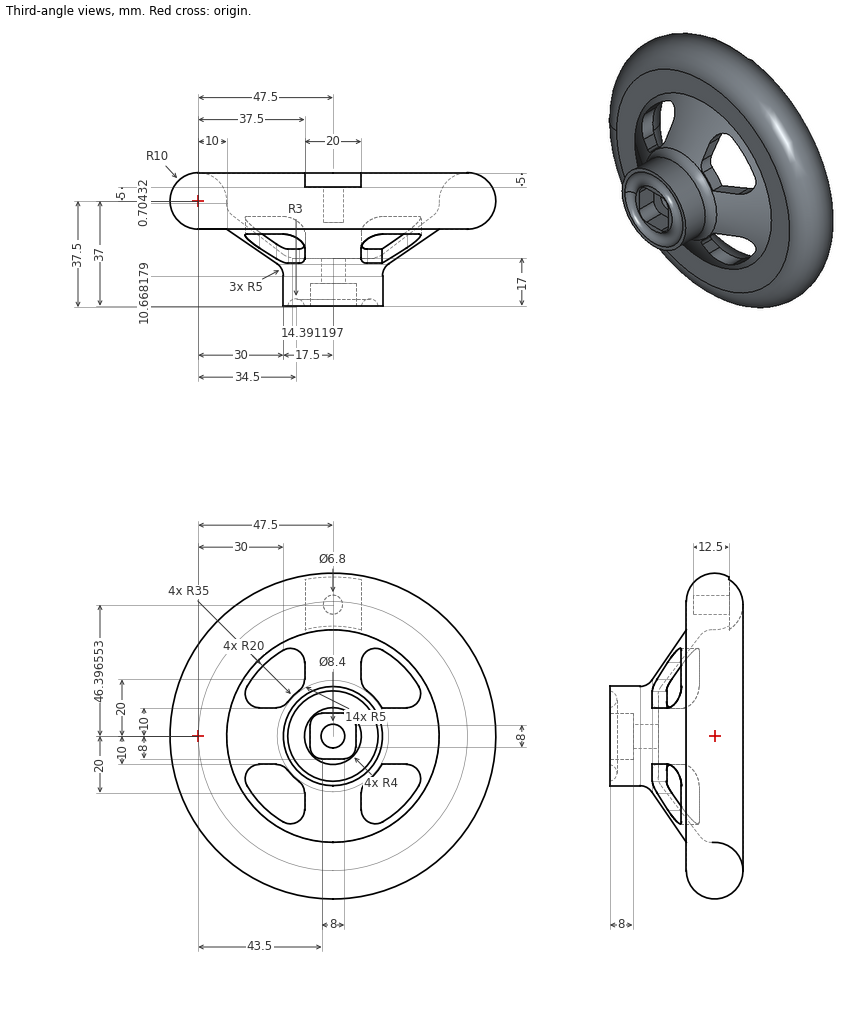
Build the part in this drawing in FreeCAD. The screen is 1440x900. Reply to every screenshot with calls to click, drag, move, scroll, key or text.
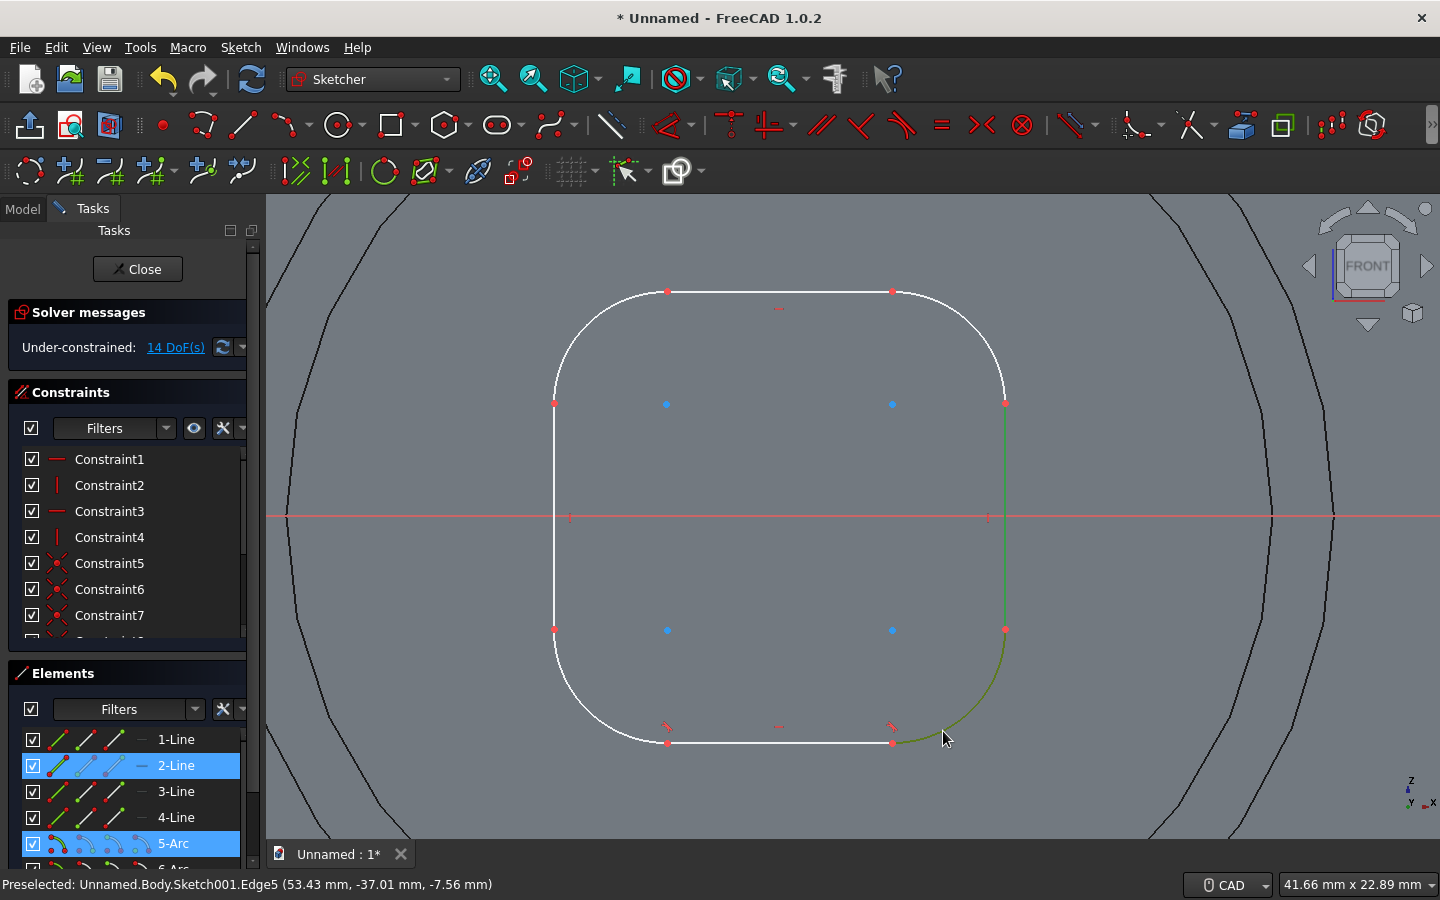
click(902, 126)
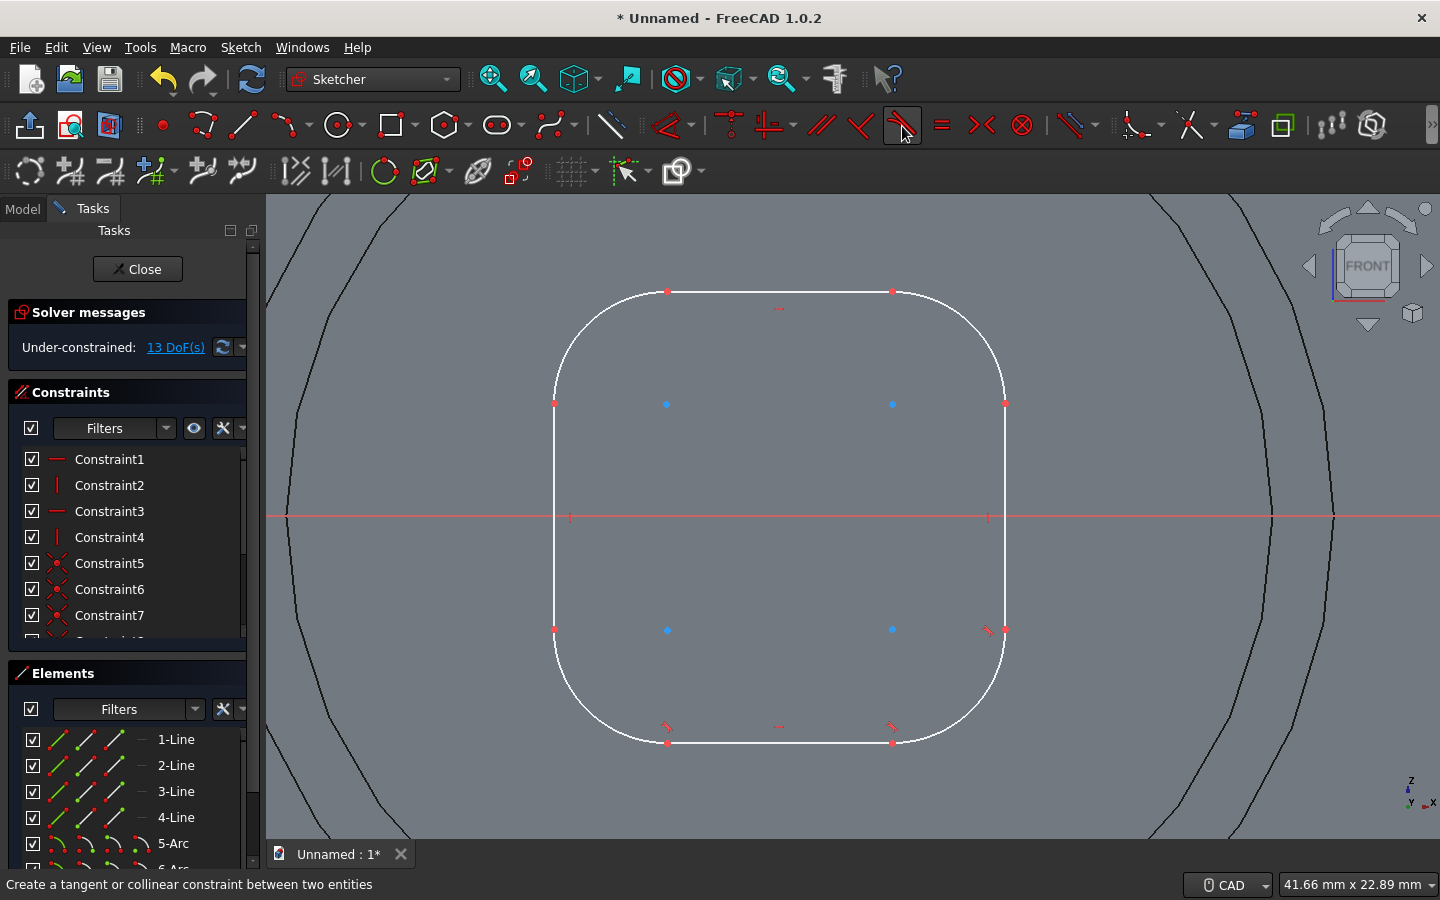
click(1005, 562)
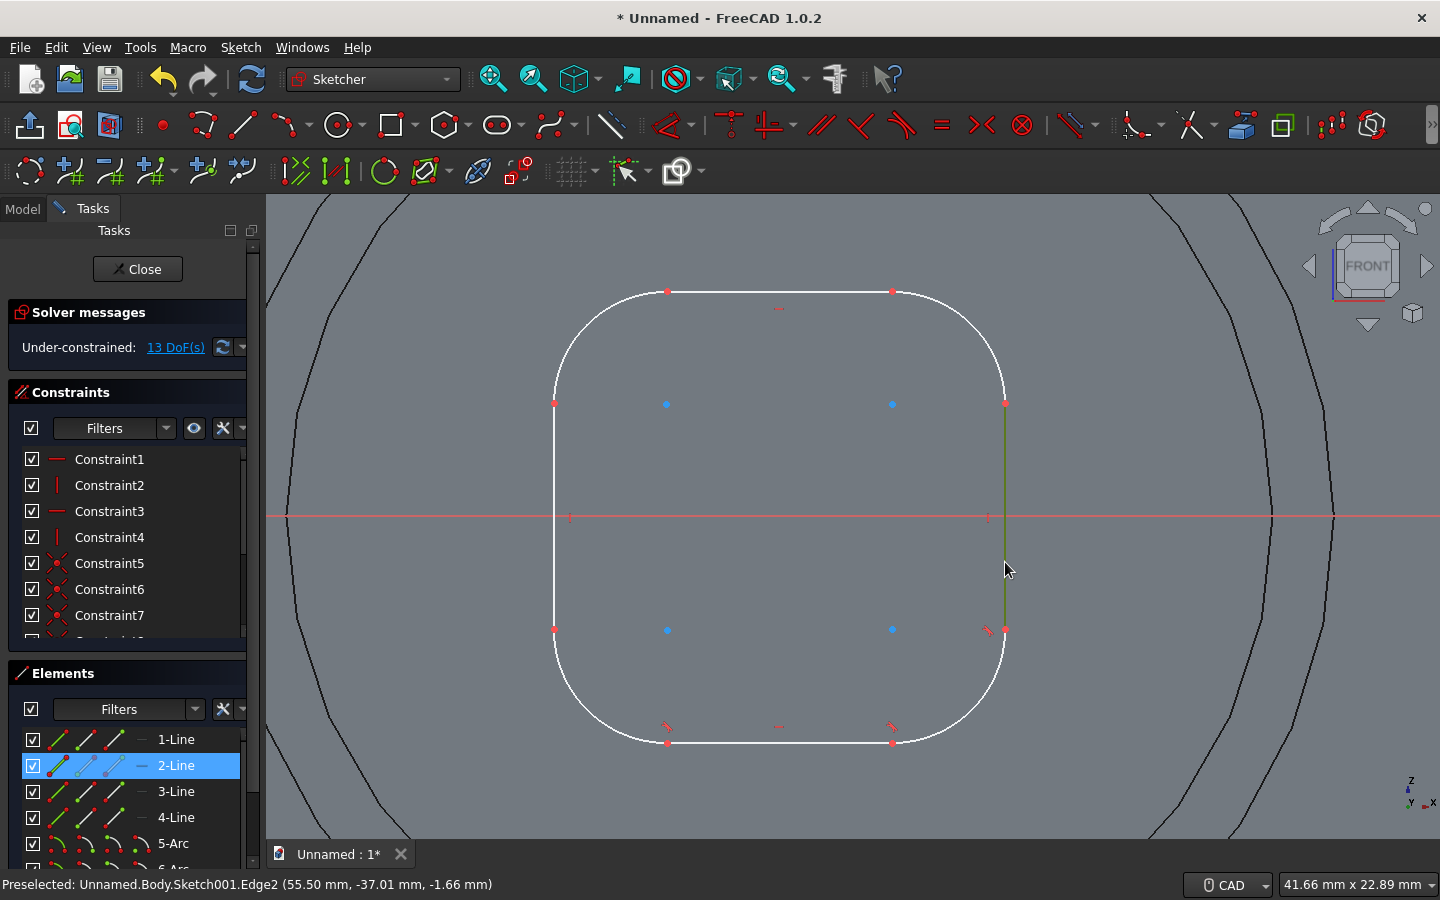
click(992, 353)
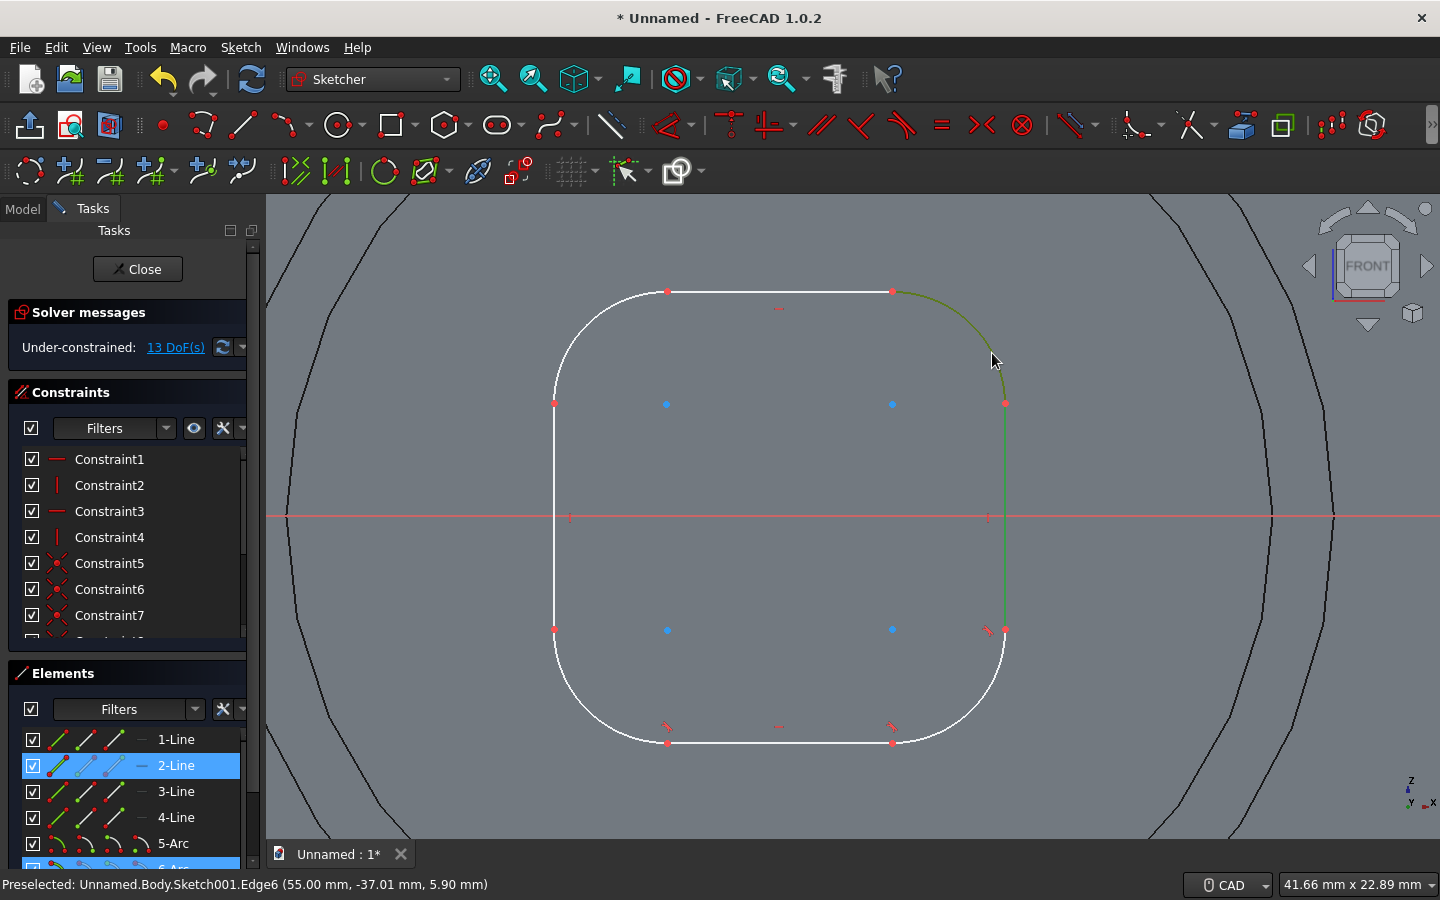
click(902, 126)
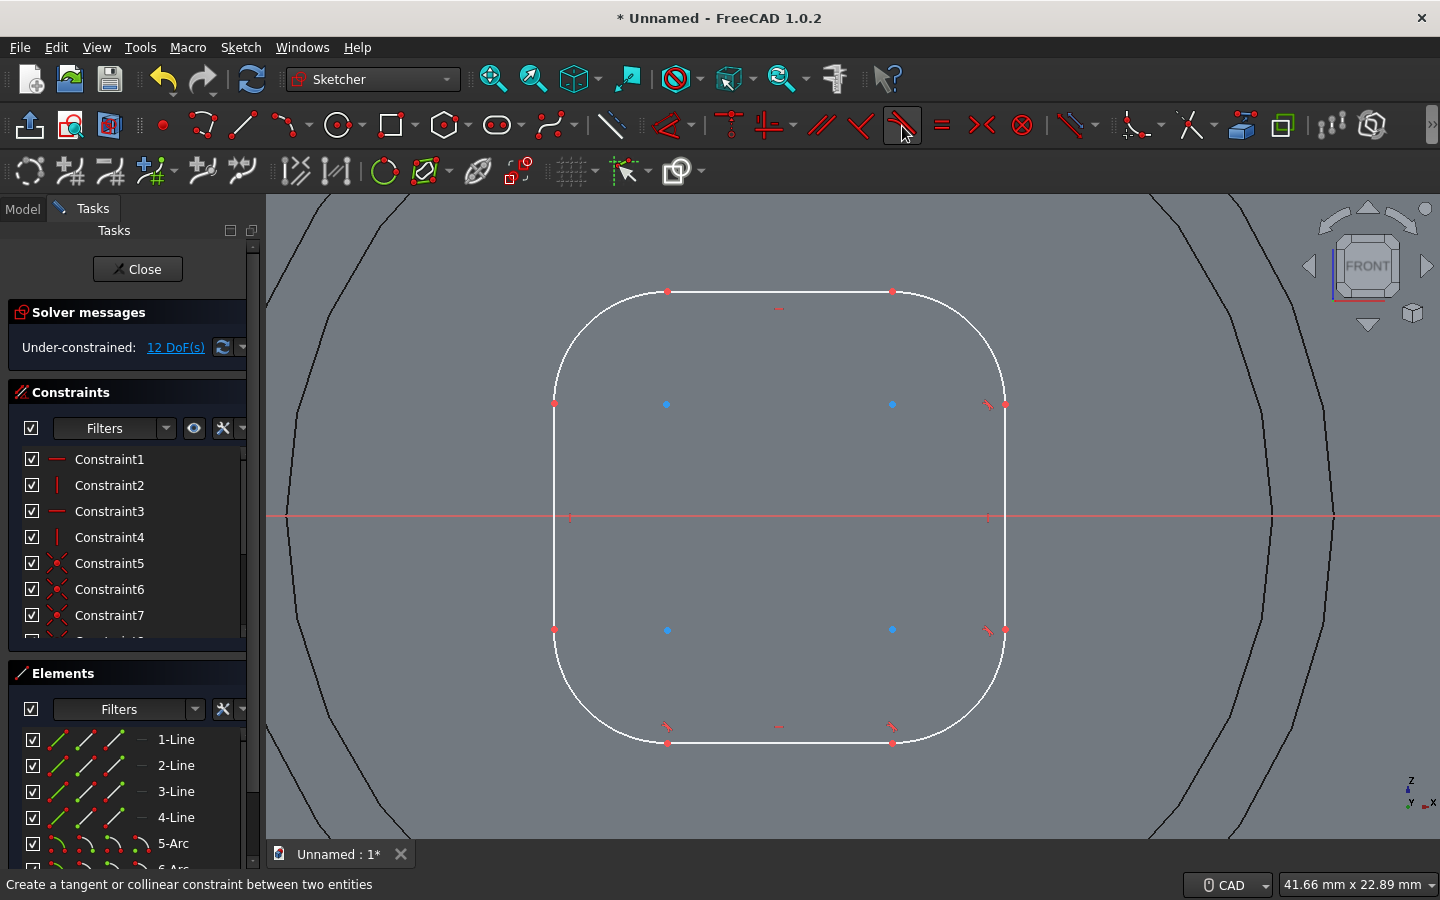
click(824, 292)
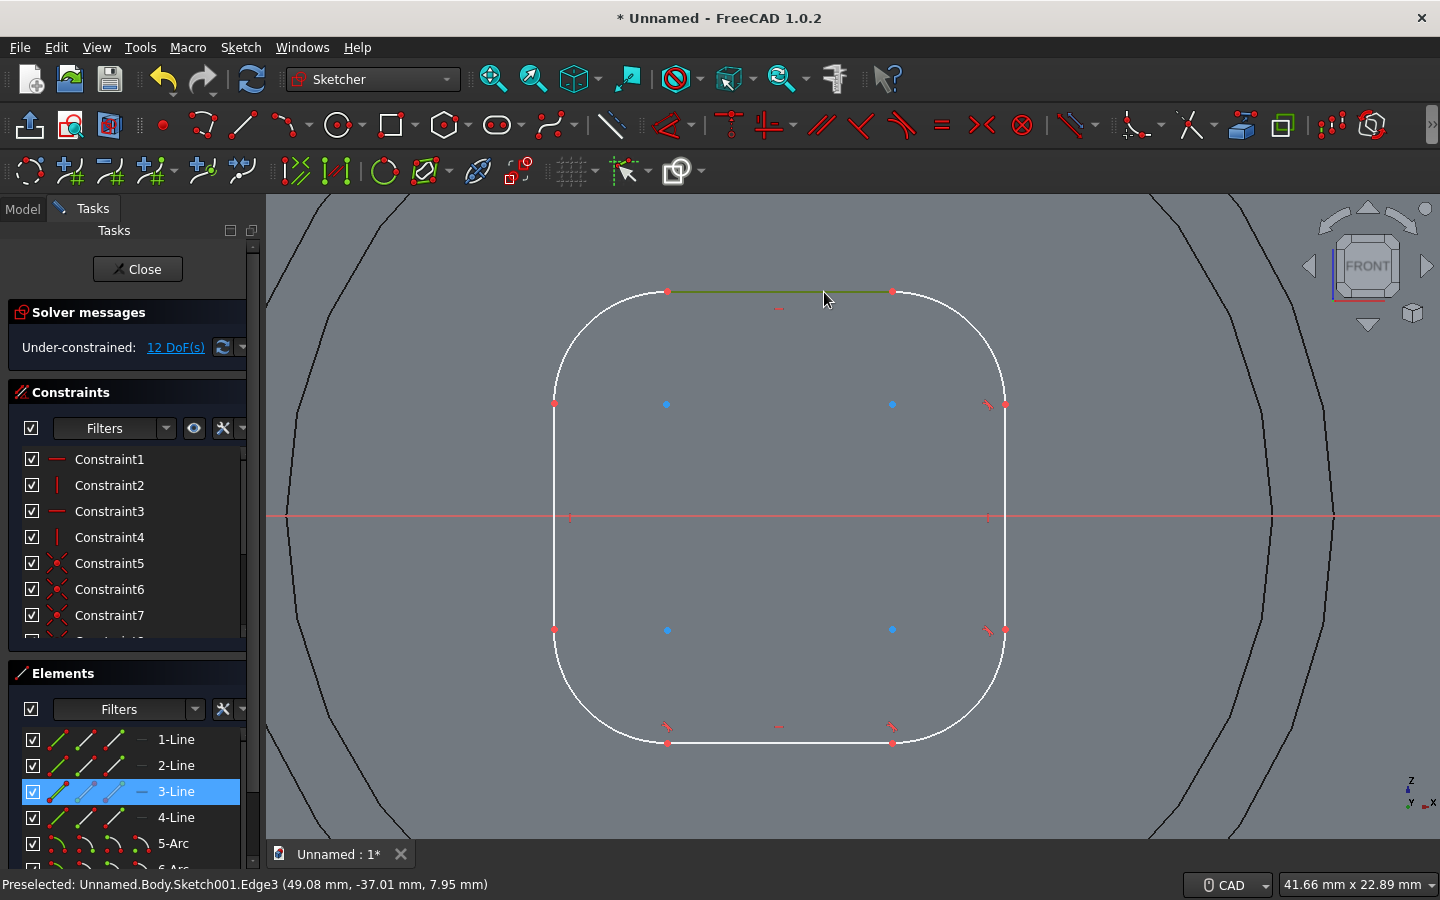
click(993, 353)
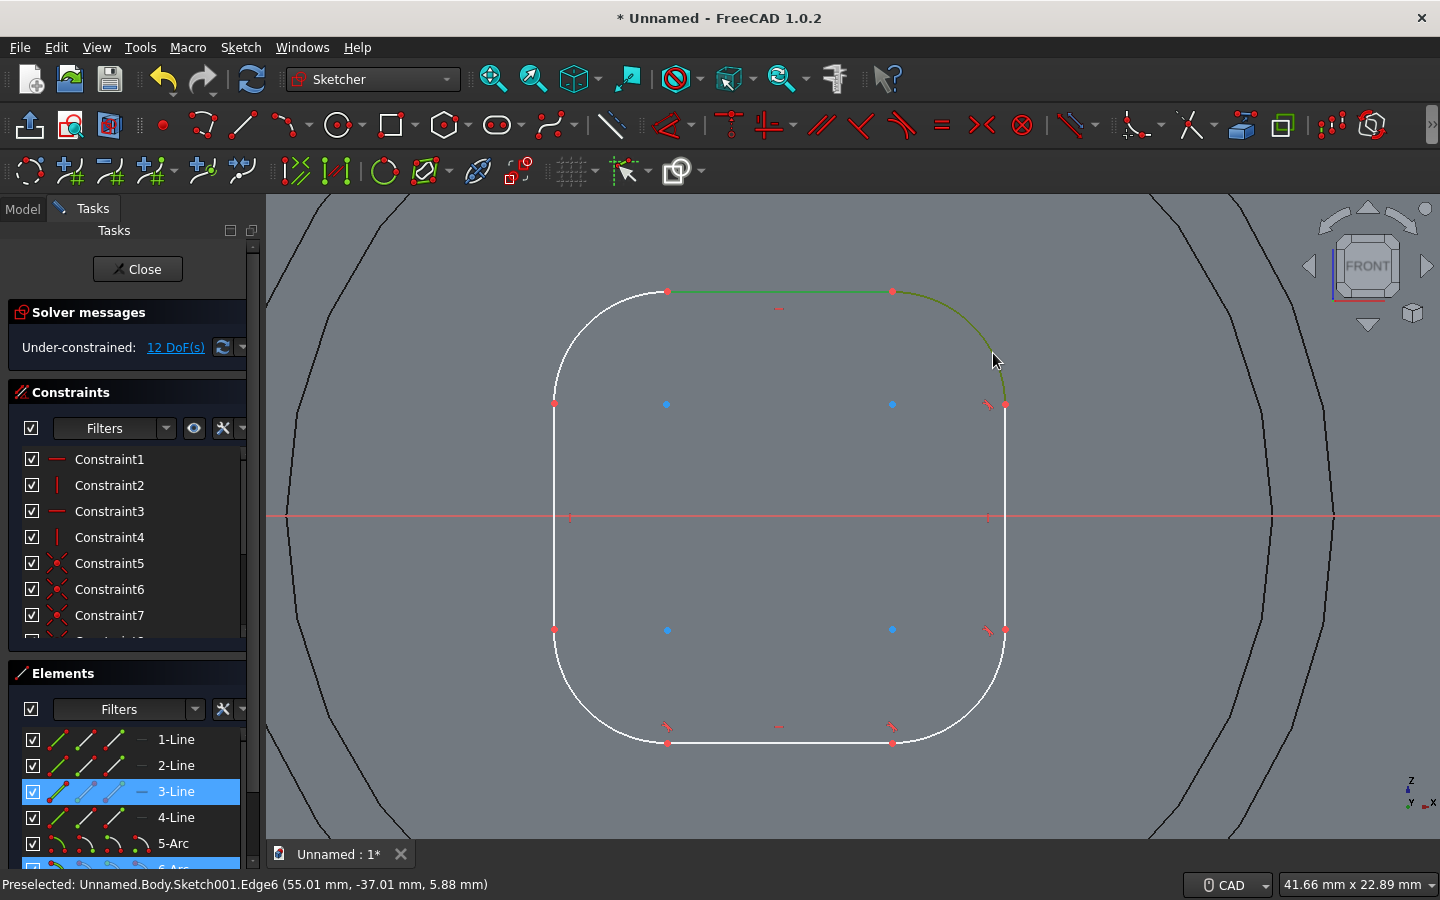
click(902, 126)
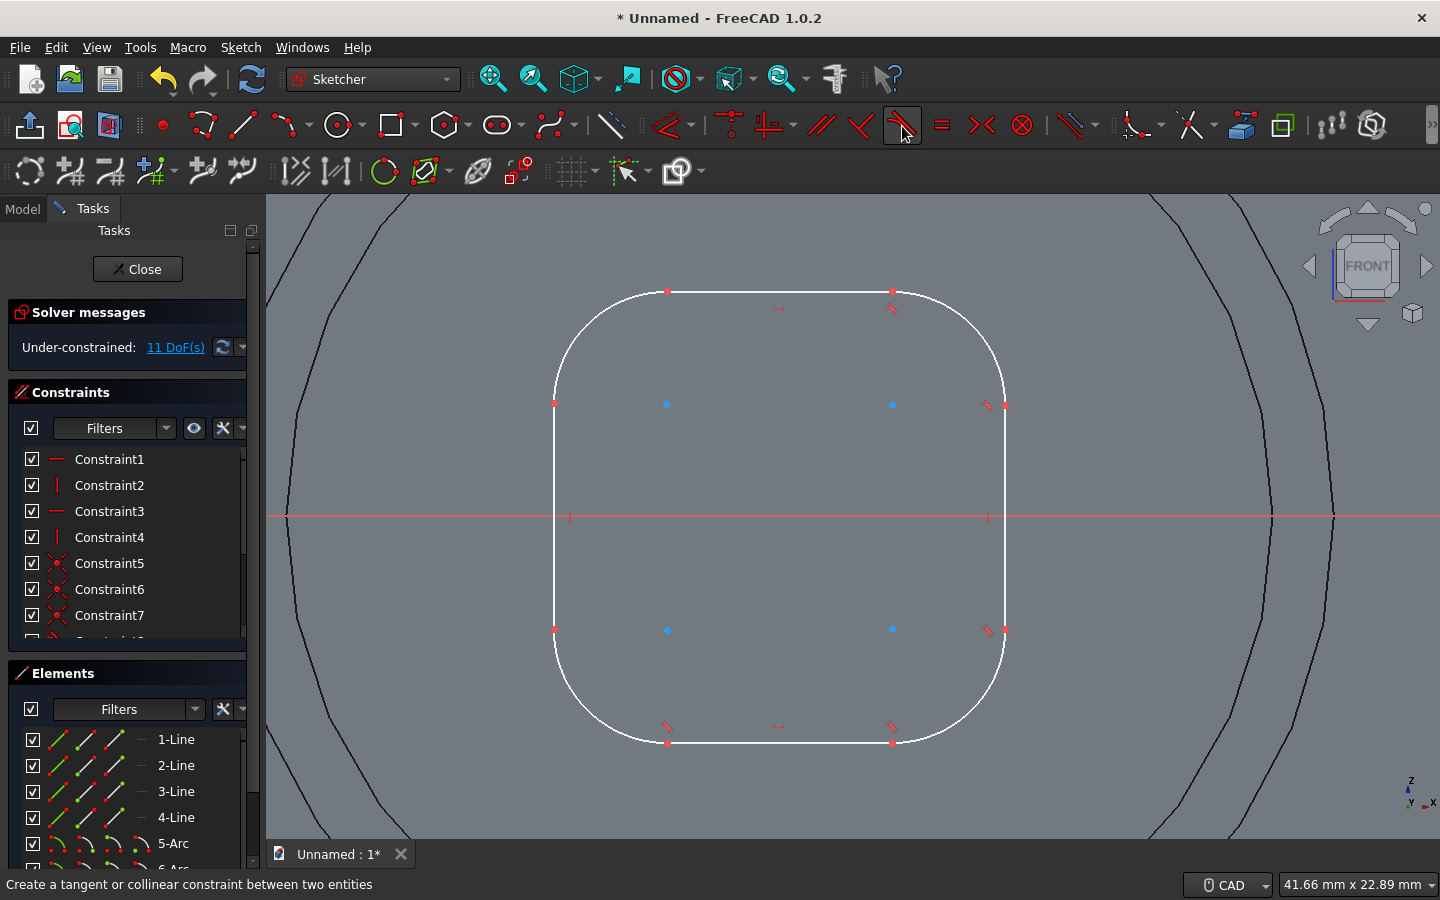
click(824, 292)